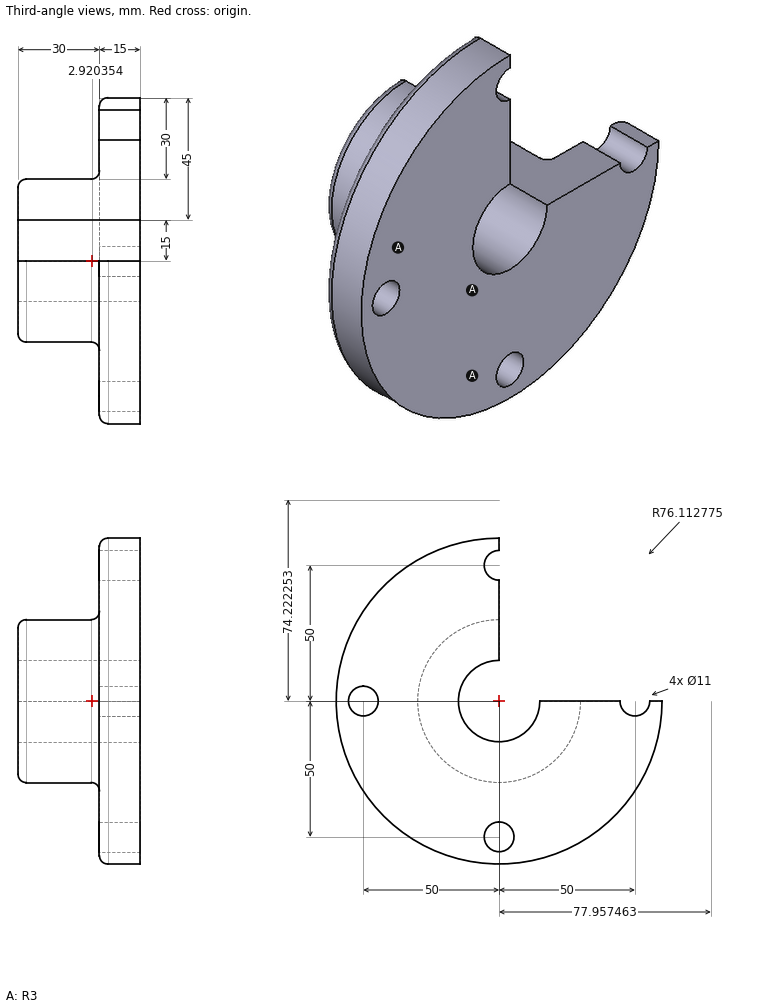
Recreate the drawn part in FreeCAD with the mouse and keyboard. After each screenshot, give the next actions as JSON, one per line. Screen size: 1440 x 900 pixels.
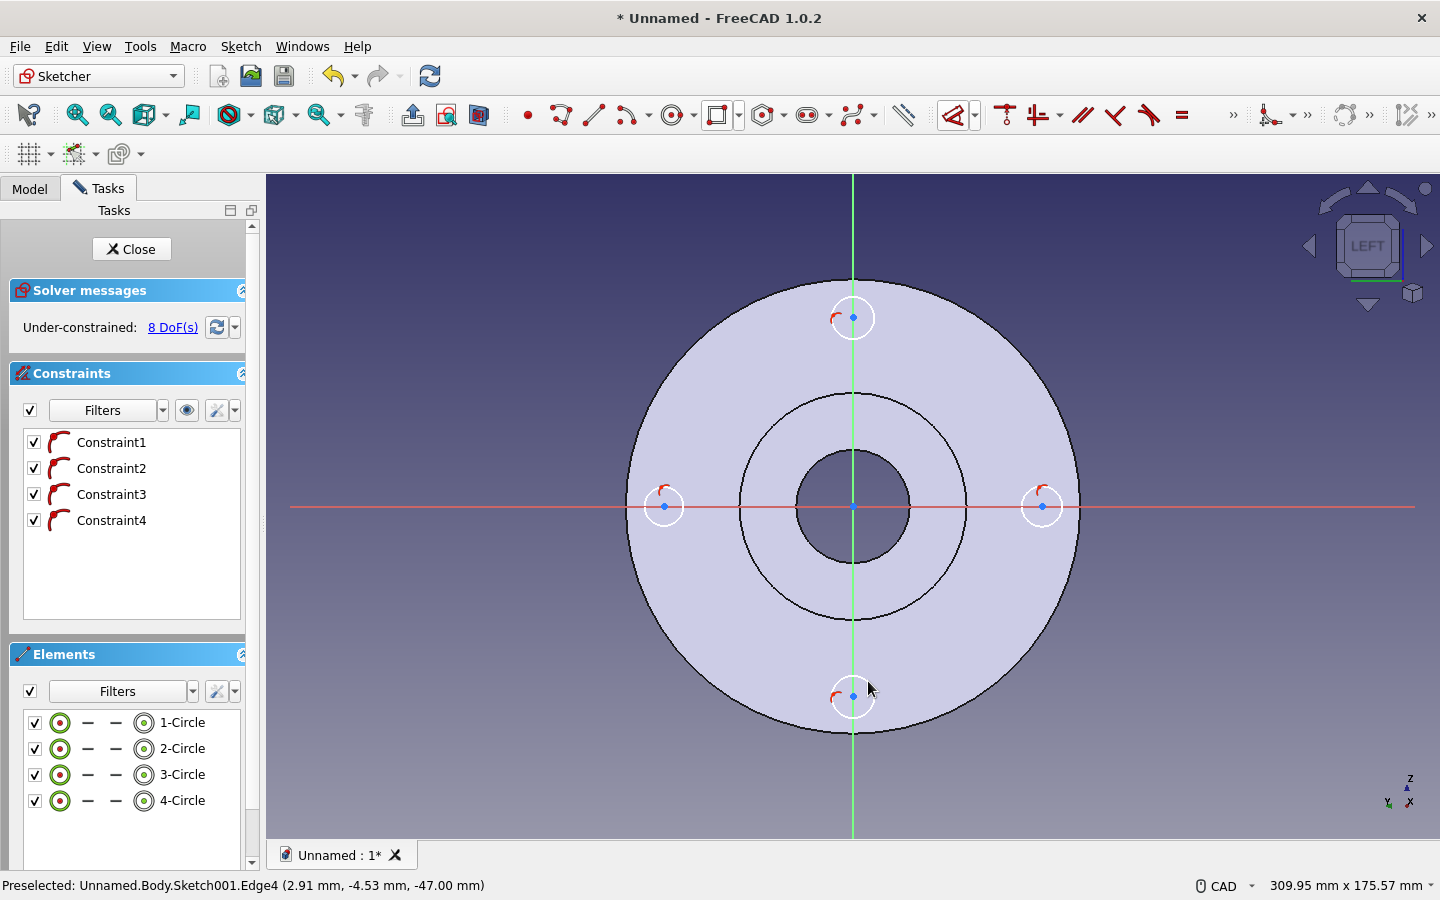
{"action": "left_click", "coordinate": [678, 493]}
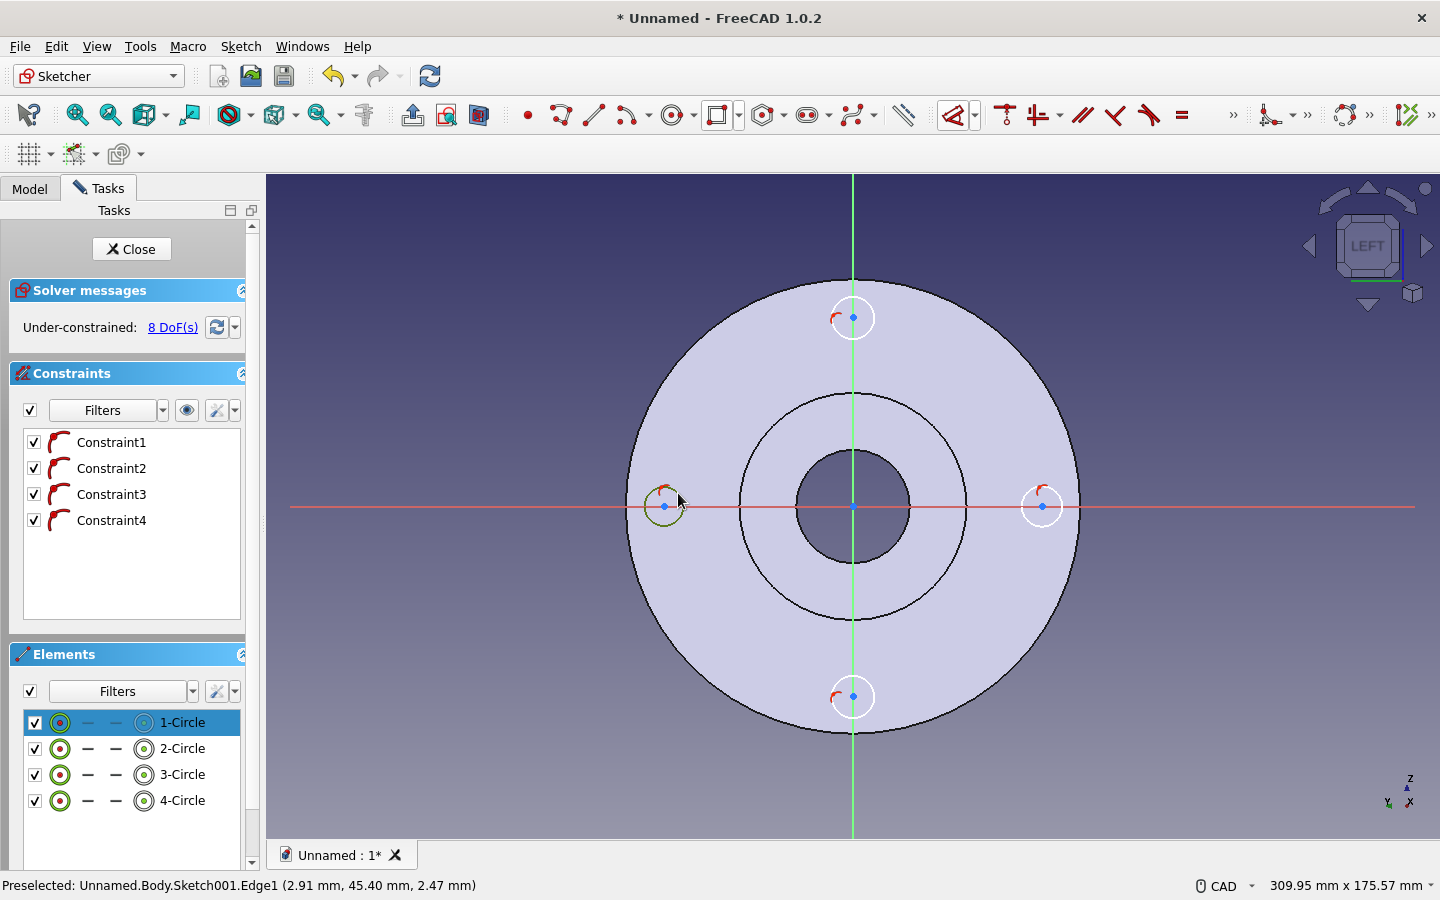
{"action": "left_click", "coordinate": [868, 303]}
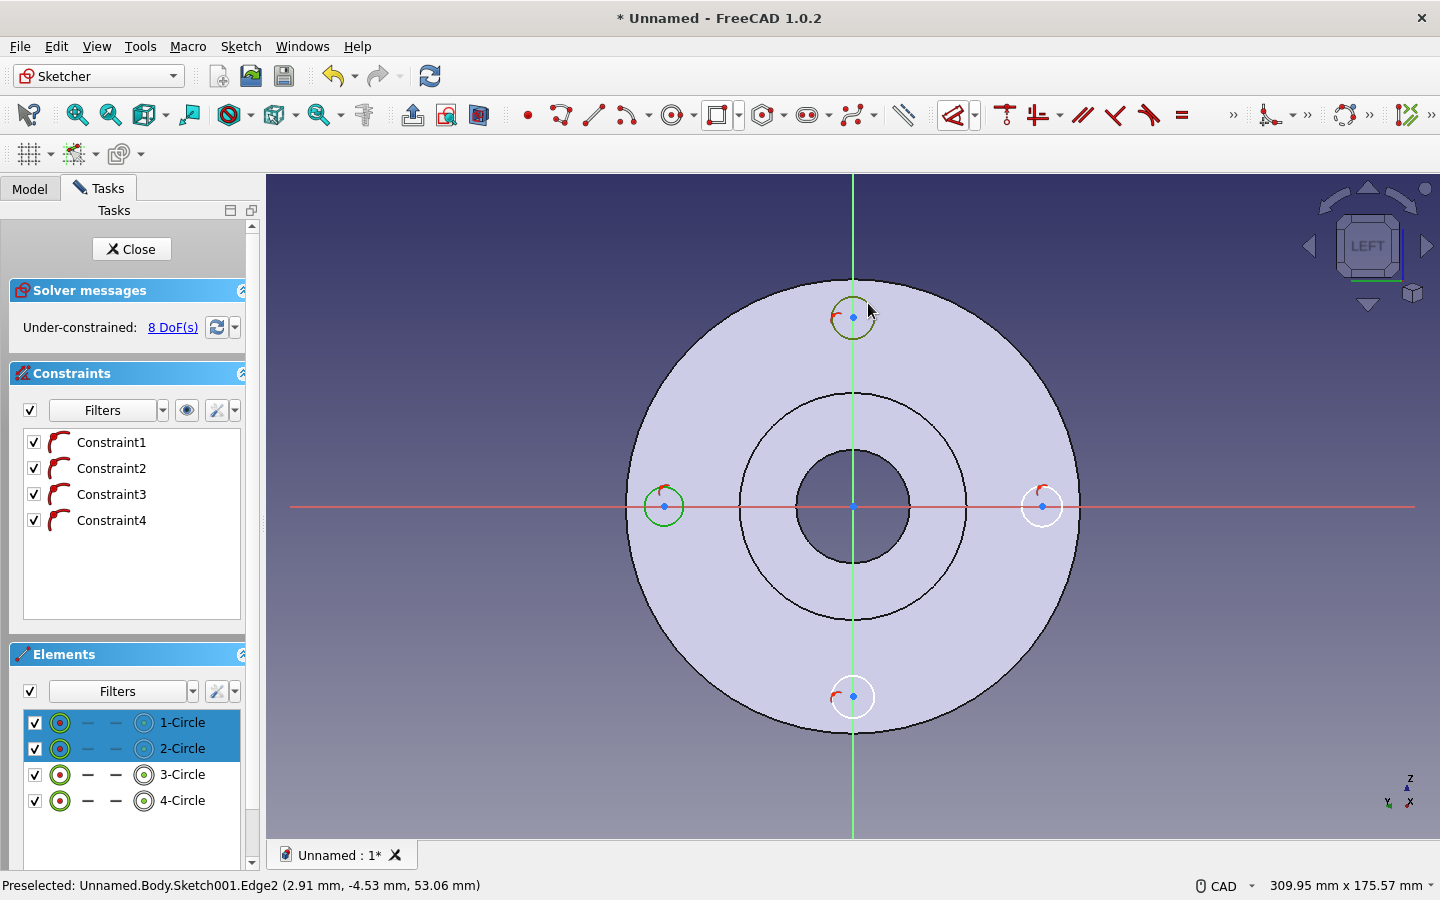
{"action": "left_click", "coordinate": [1056, 492]}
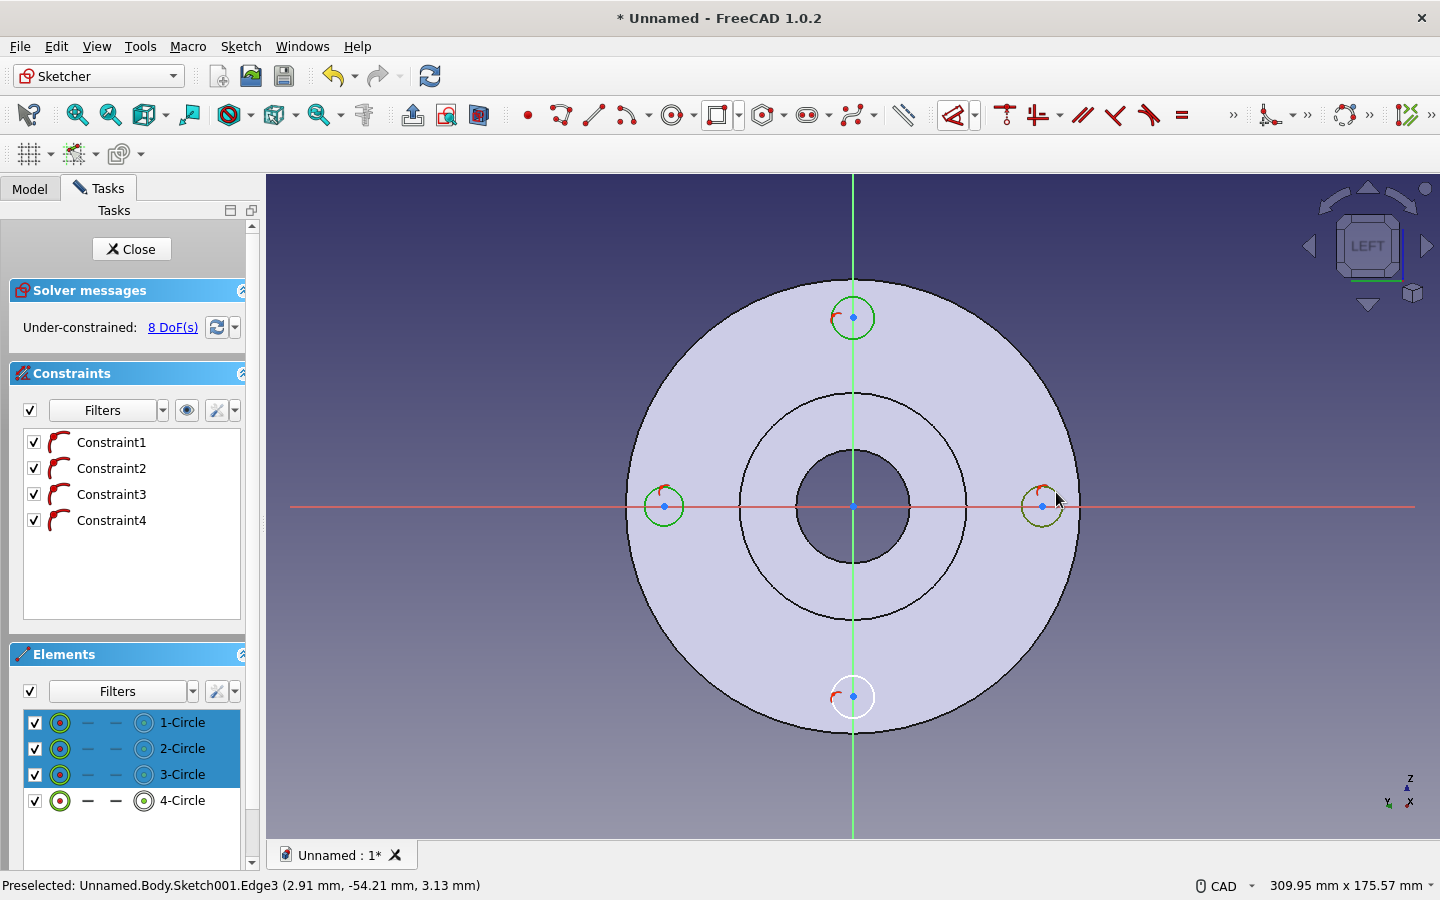
{"action": "left_click", "coordinate": [868, 682]}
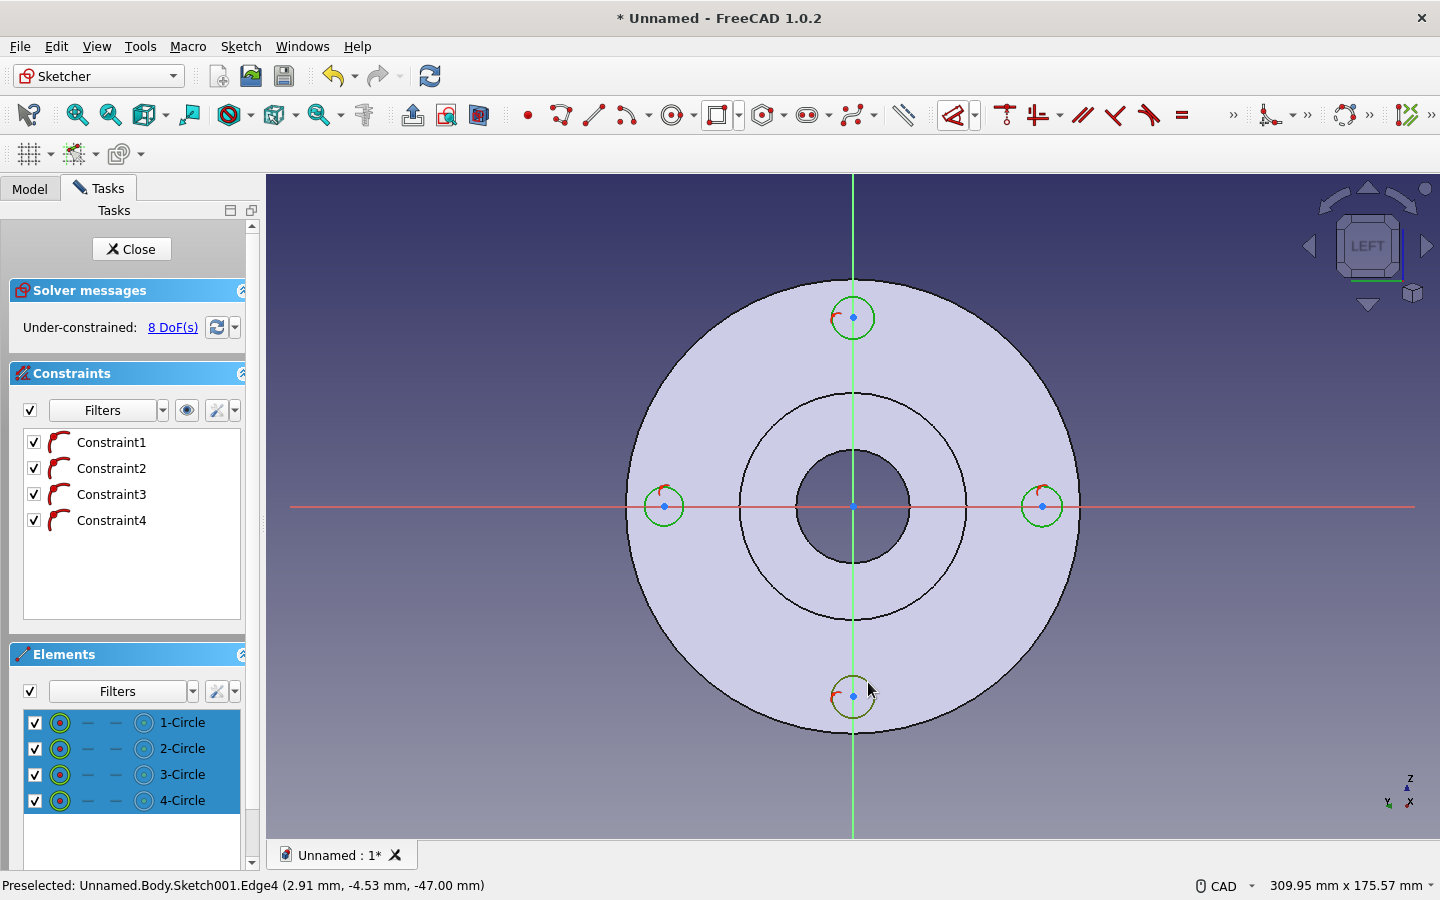
{"action": "left_click", "coordinate": [1182, 116]}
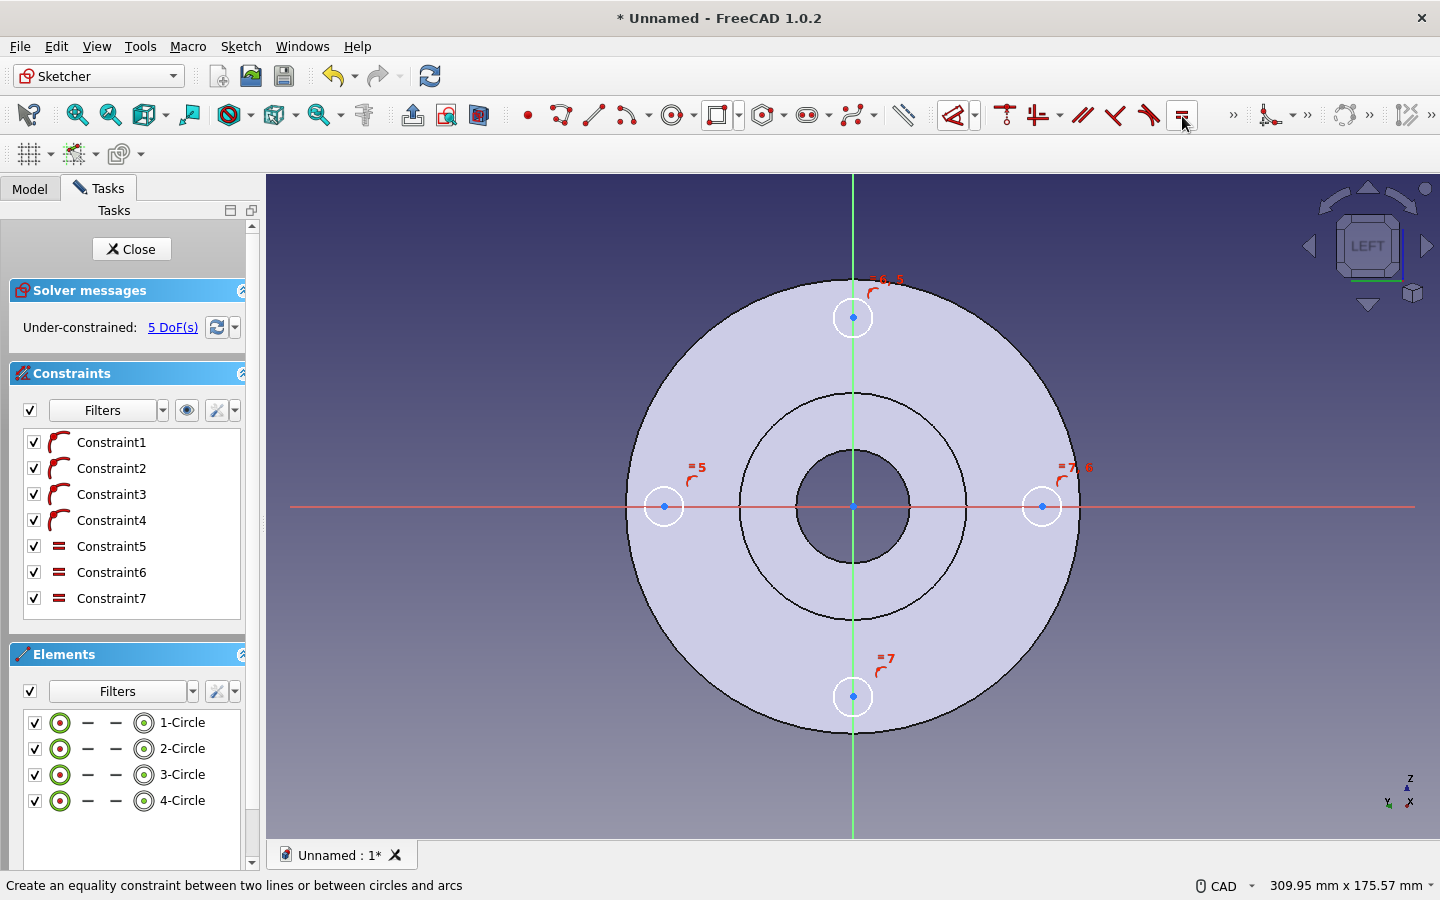
{"action": "left_click", "coordinate": [678, 493]}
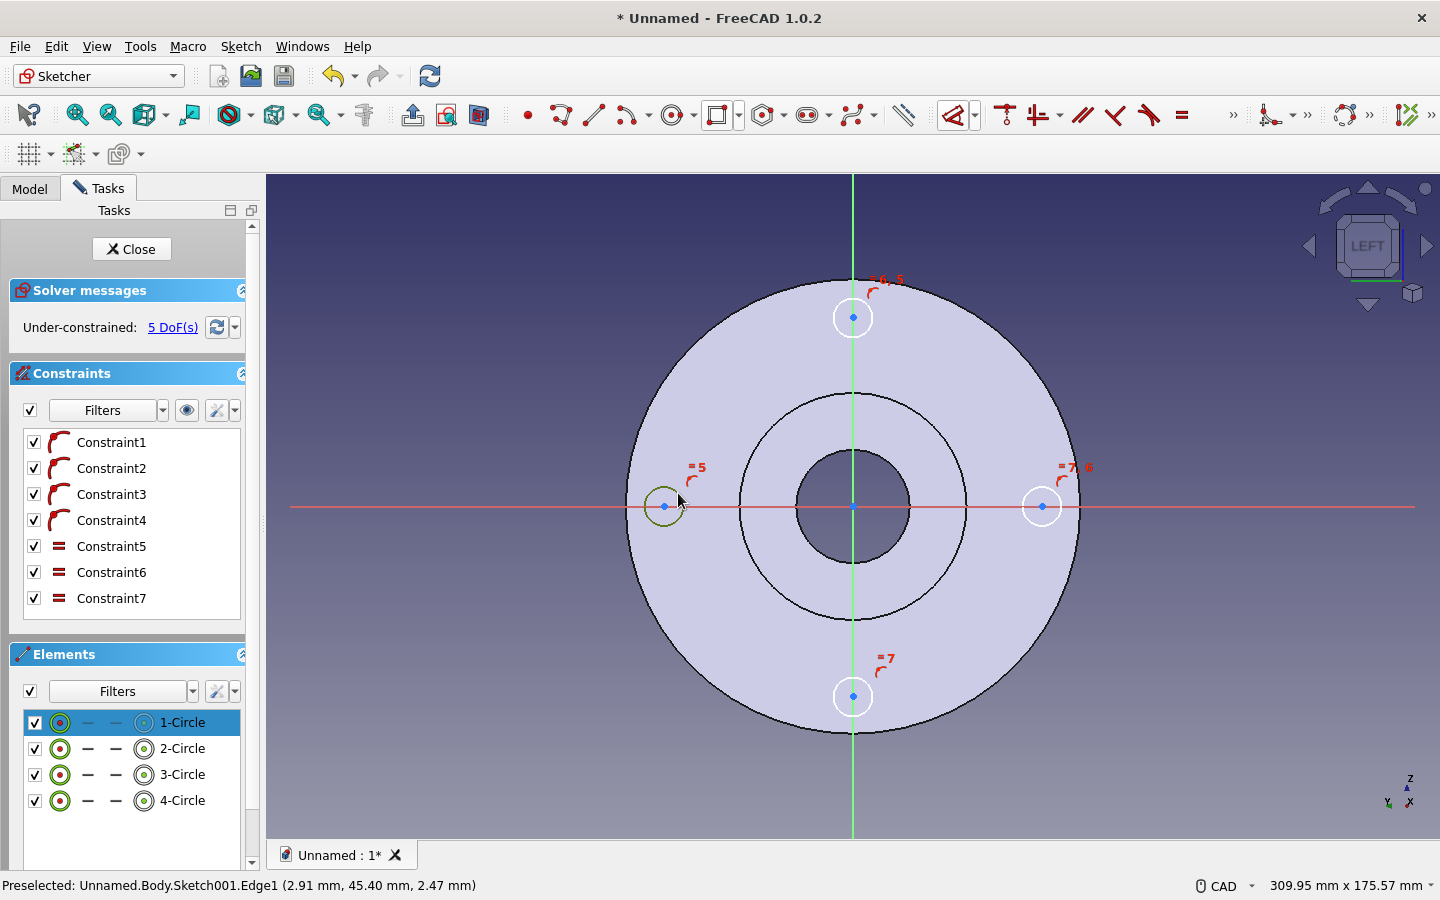
{"action": "key", "text": "k o"}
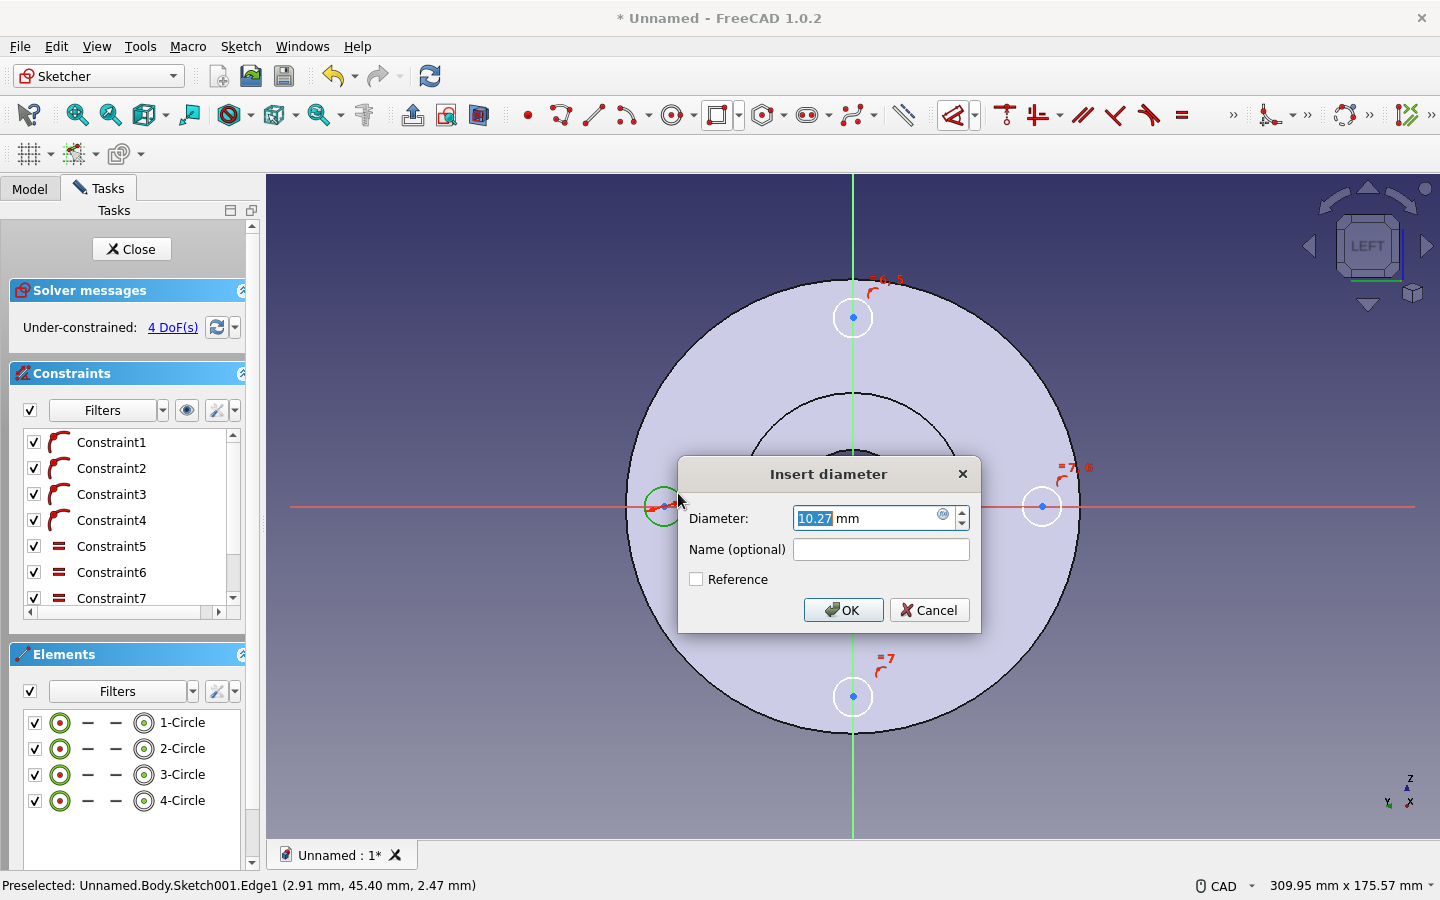
{"action": "type", "text": "11"}
{"action": "key", "text": "Return"}